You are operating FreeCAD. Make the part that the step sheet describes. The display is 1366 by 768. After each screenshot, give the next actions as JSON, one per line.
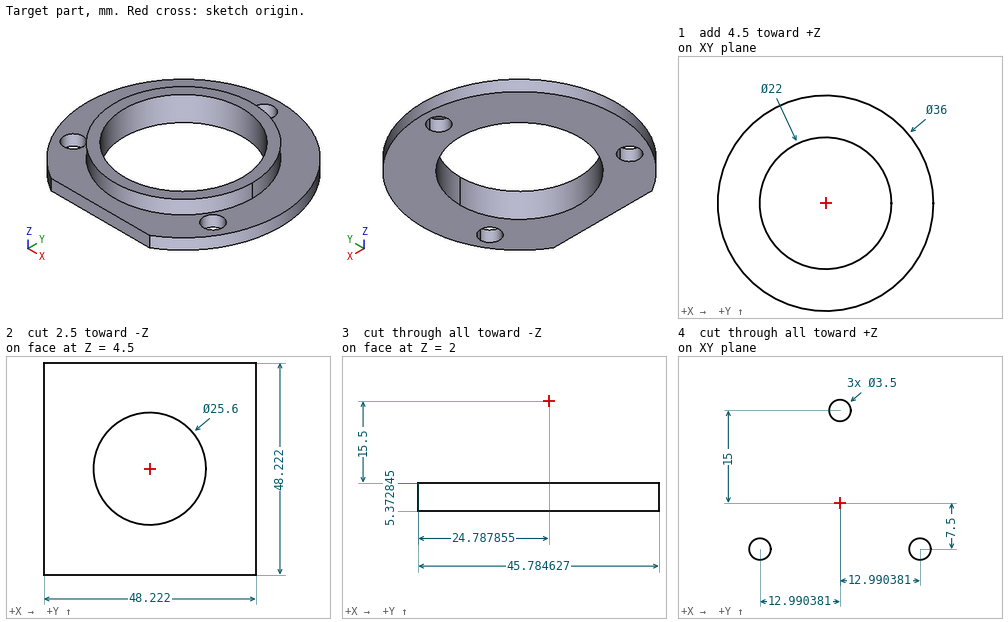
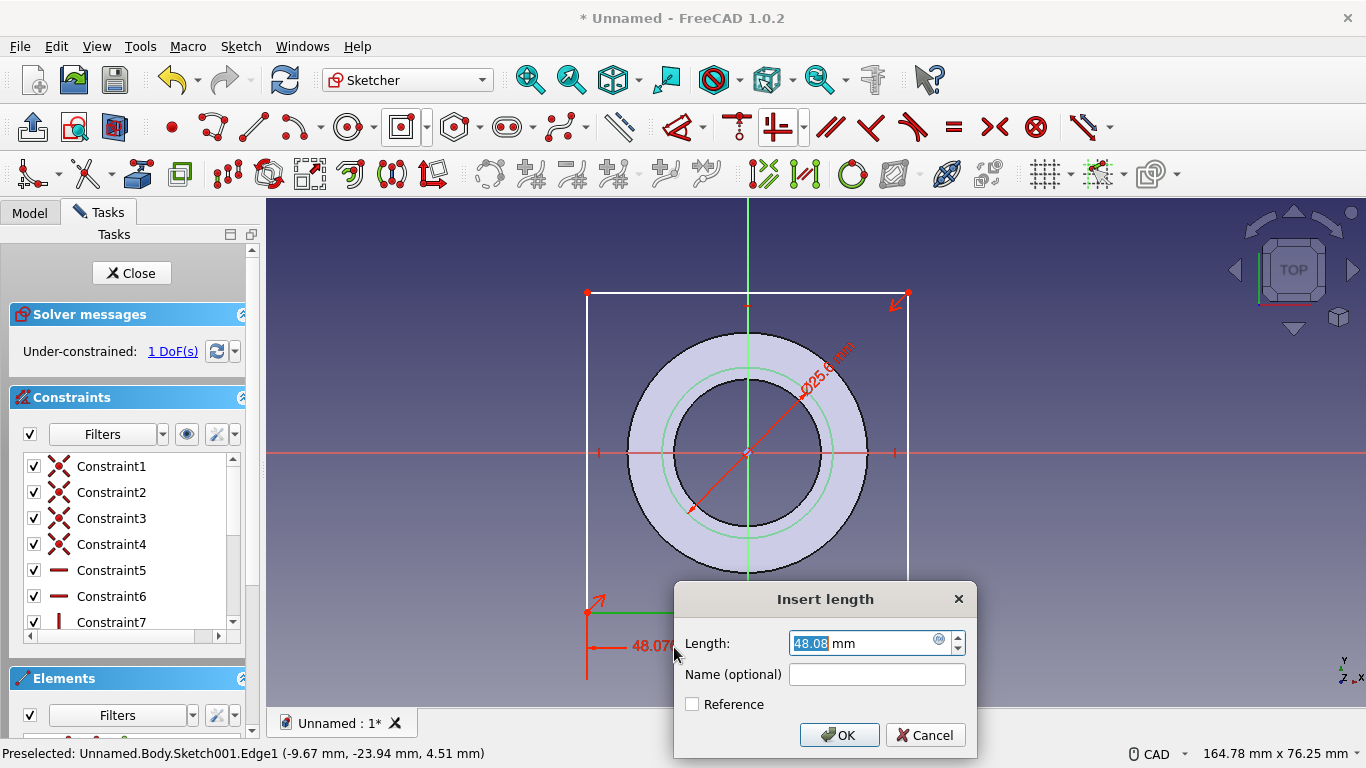
{"action": "type", "text": "48.222"}
{"action": "key", "text": "Return"}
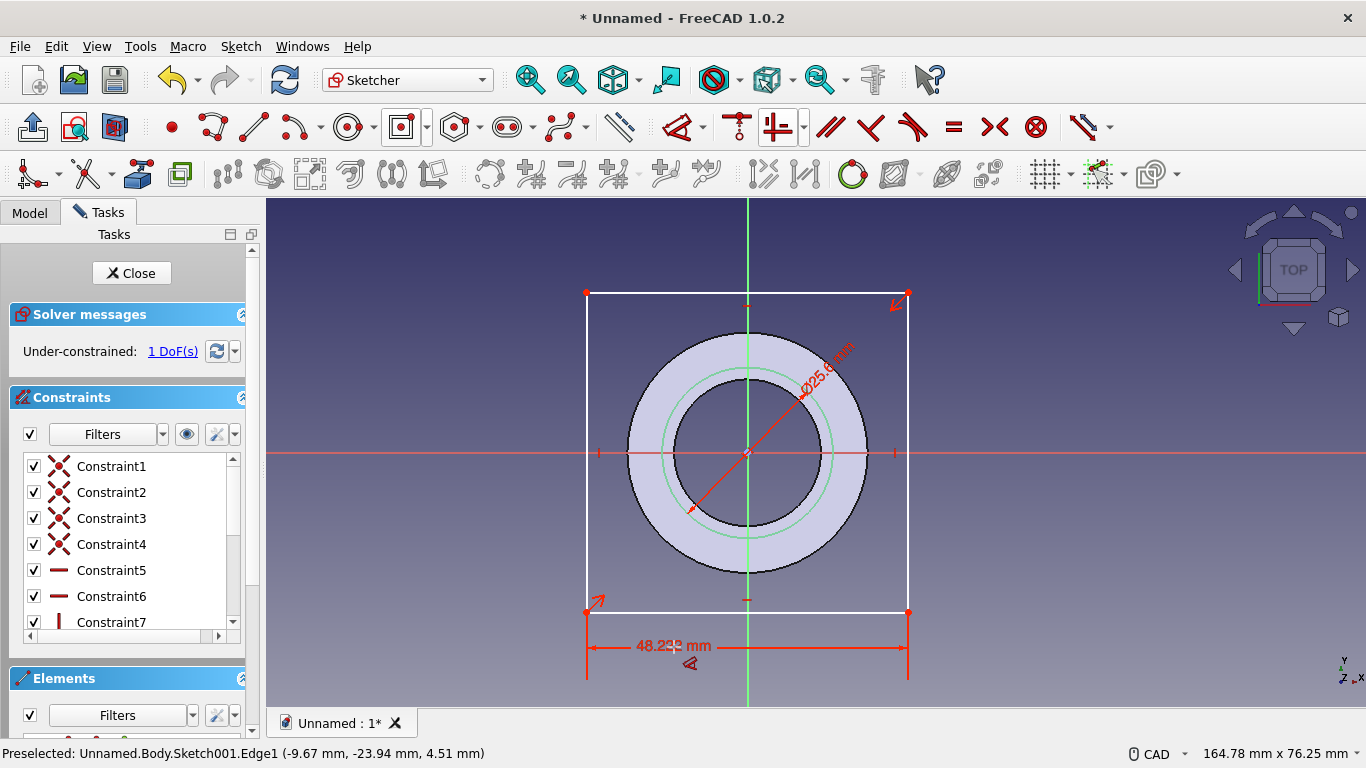
{"action": "left_click", "coordinate": [908, 517]}
{"action": "left_click", "coordinate": [942, 379]}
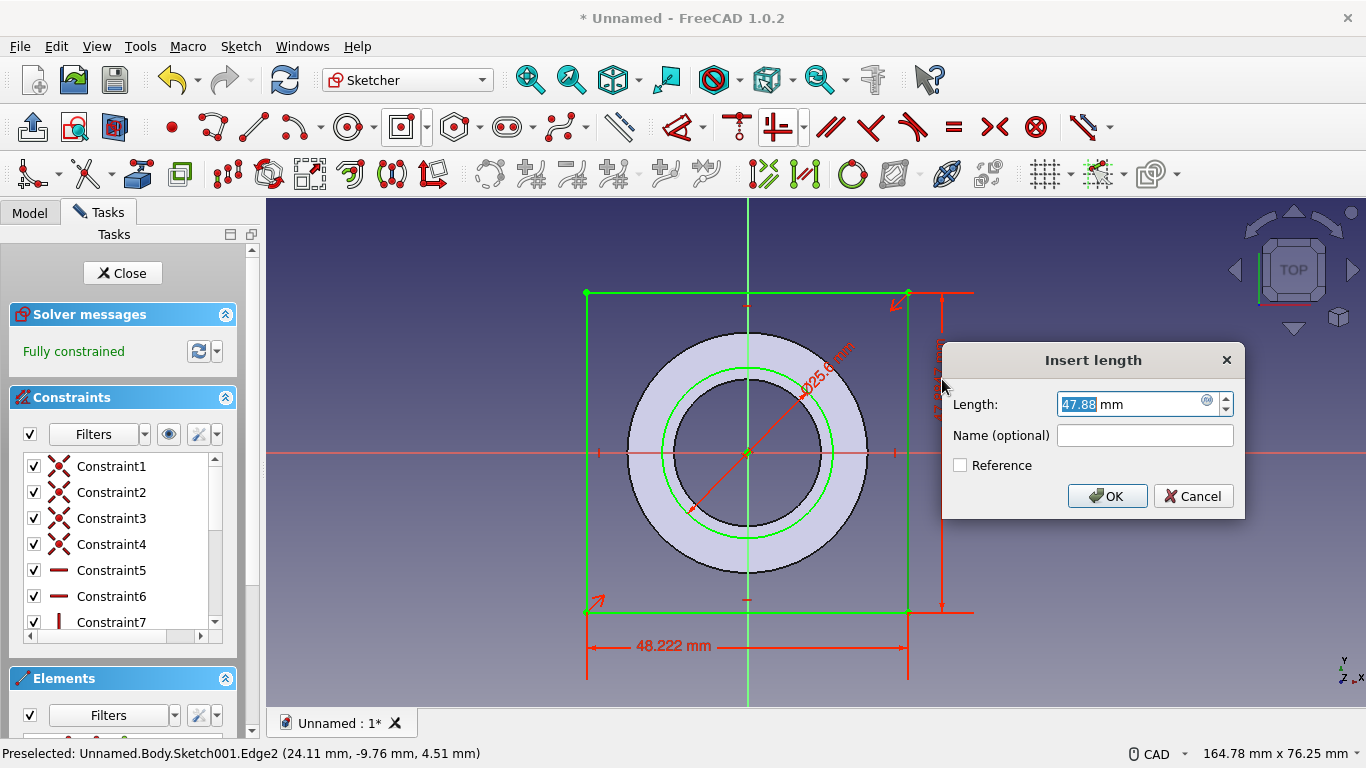
{"action": "type", "text": "48.222"}
{"action": "key", "text": "Return"}
{"action": "key", "text": "Escape"}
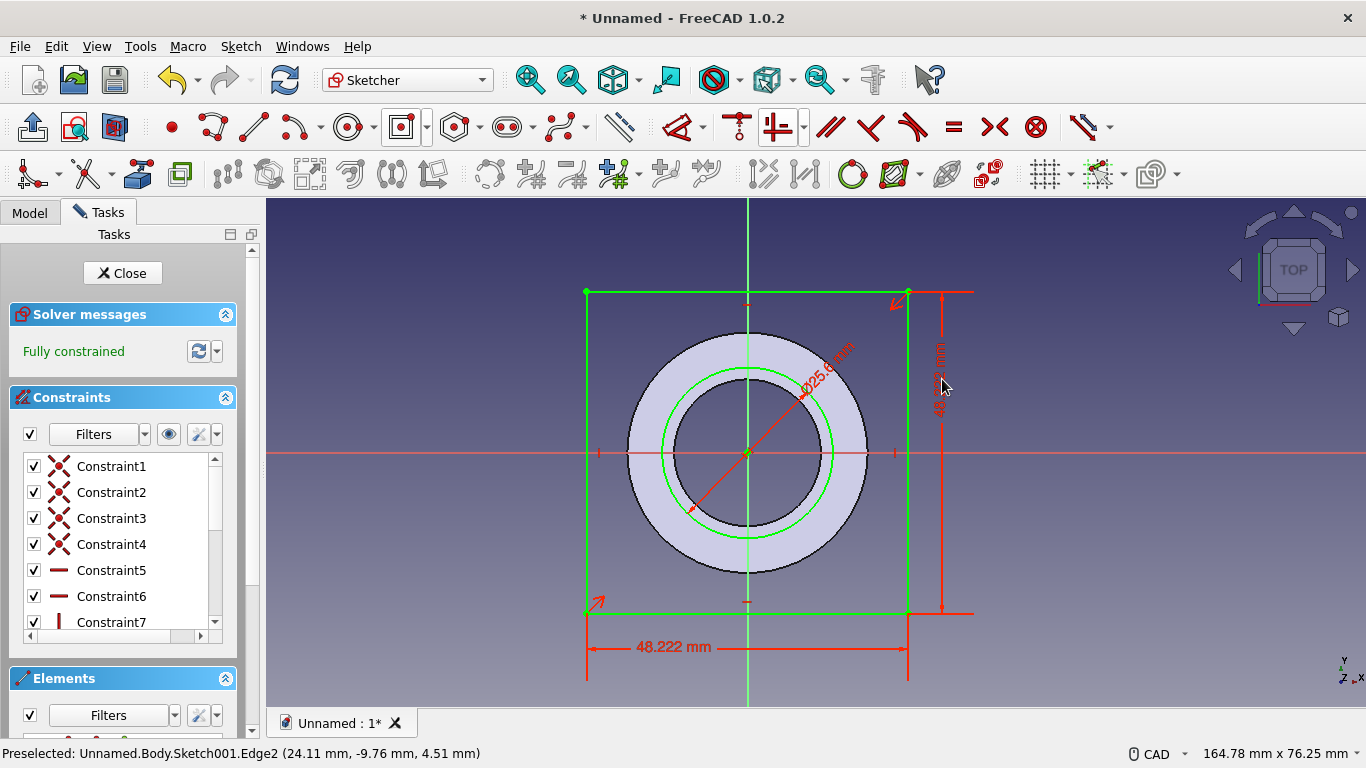
{"action": "left_click", "coordinate": [123, 273]}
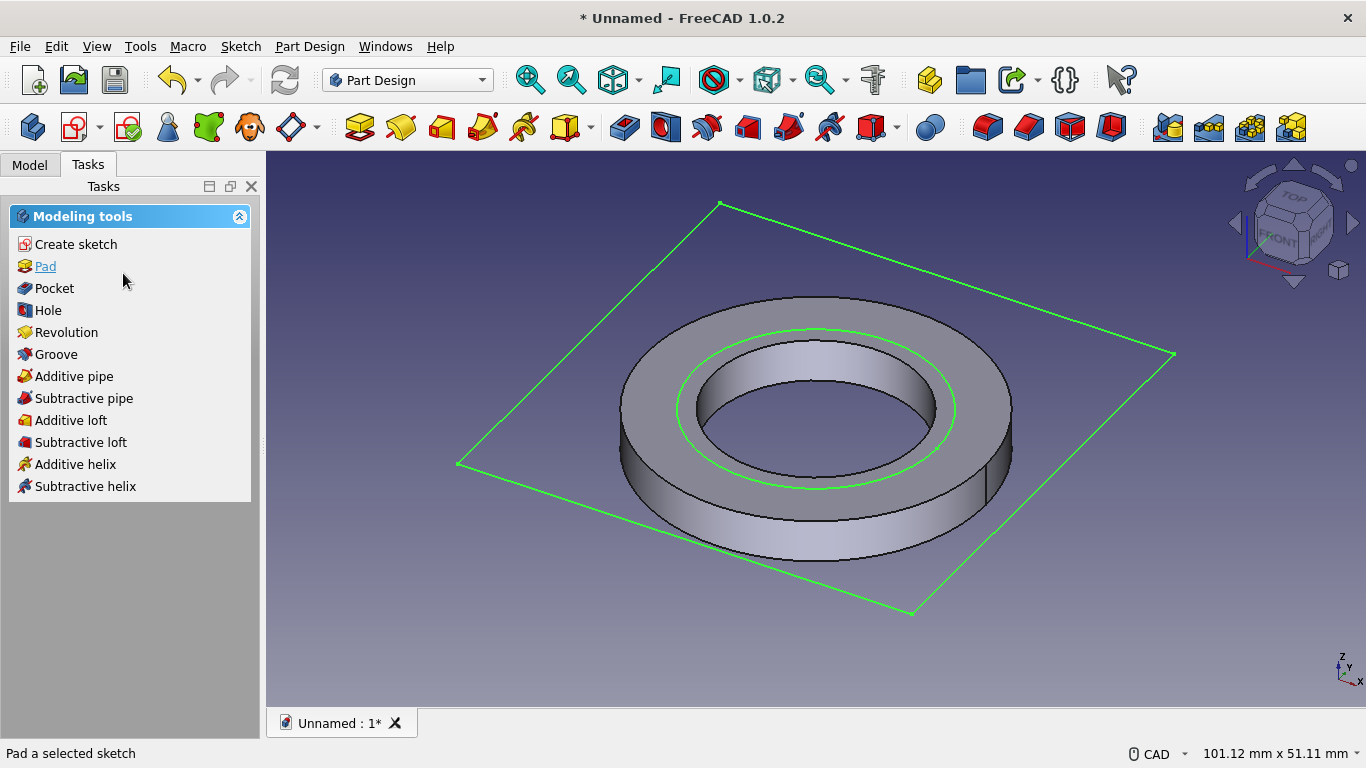
{"action": "left_click", "coordinate": [625, 128]}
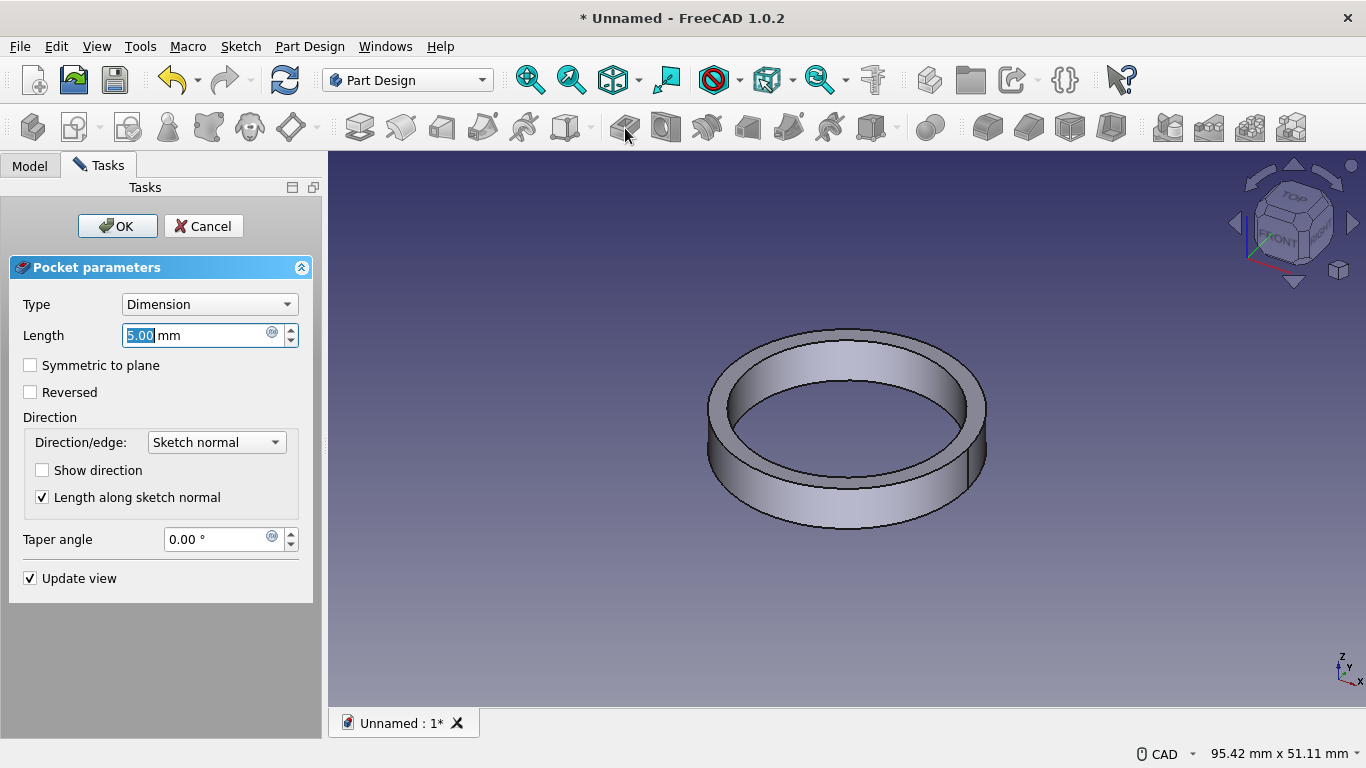
{"action": "type", "text": "2.5"}
{"action": "key", "text": "Tab"}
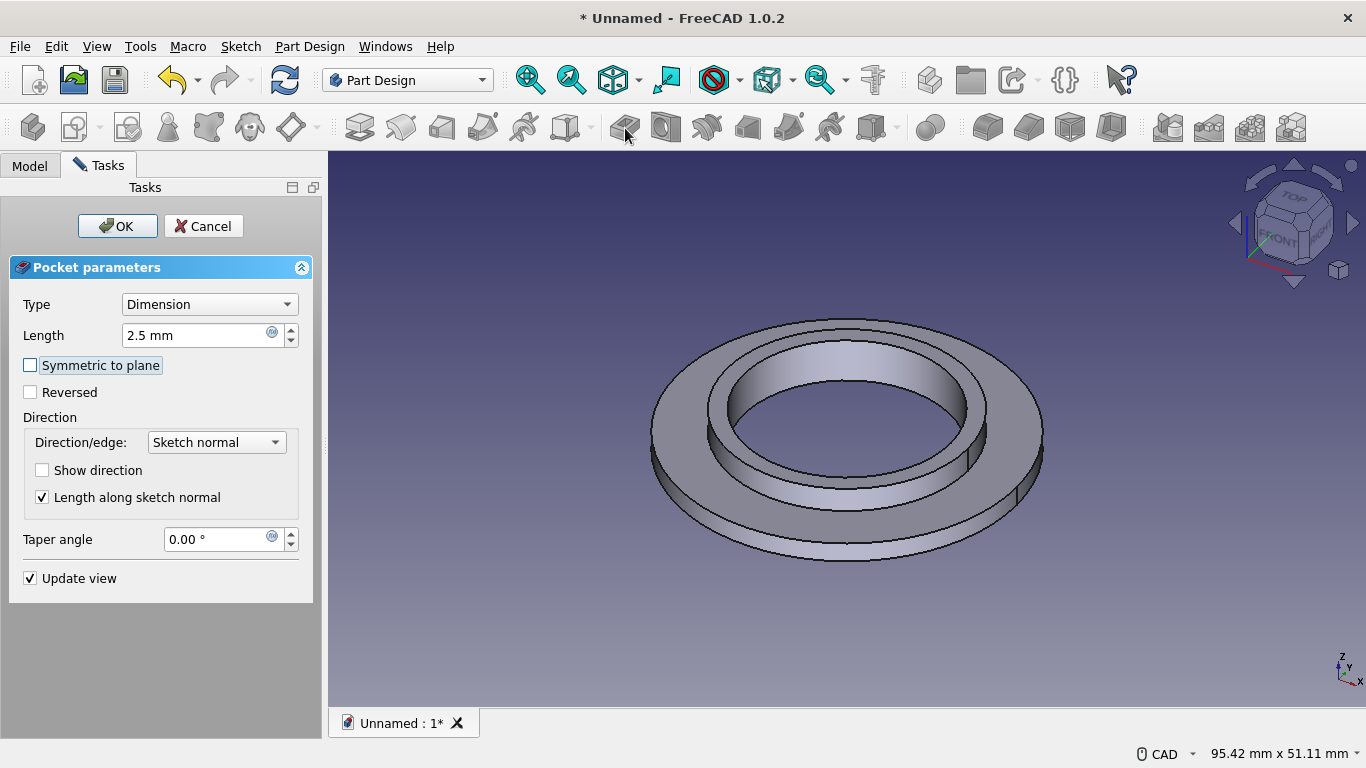
{"action": "left_click", "coordinate": [118, 226]}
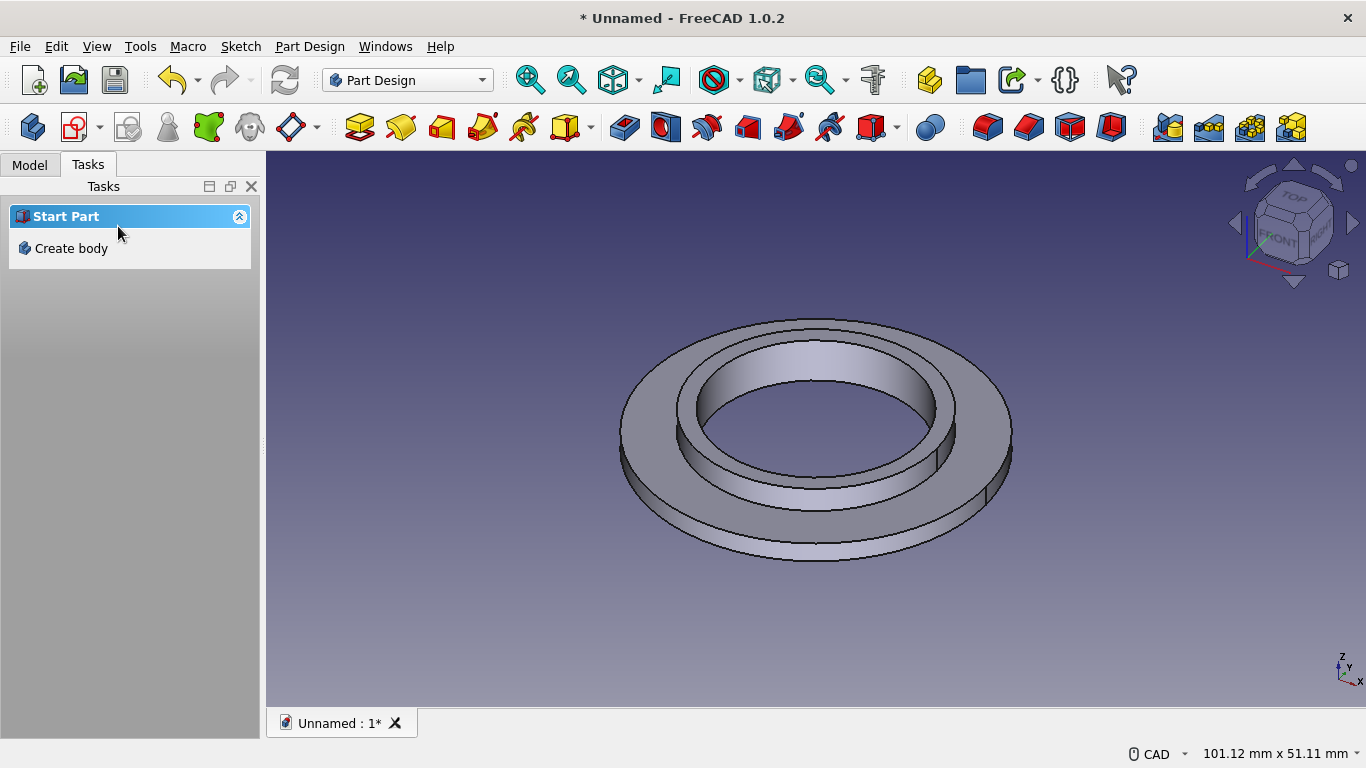
{"action": "left_click", "coordinate": [732, 514]}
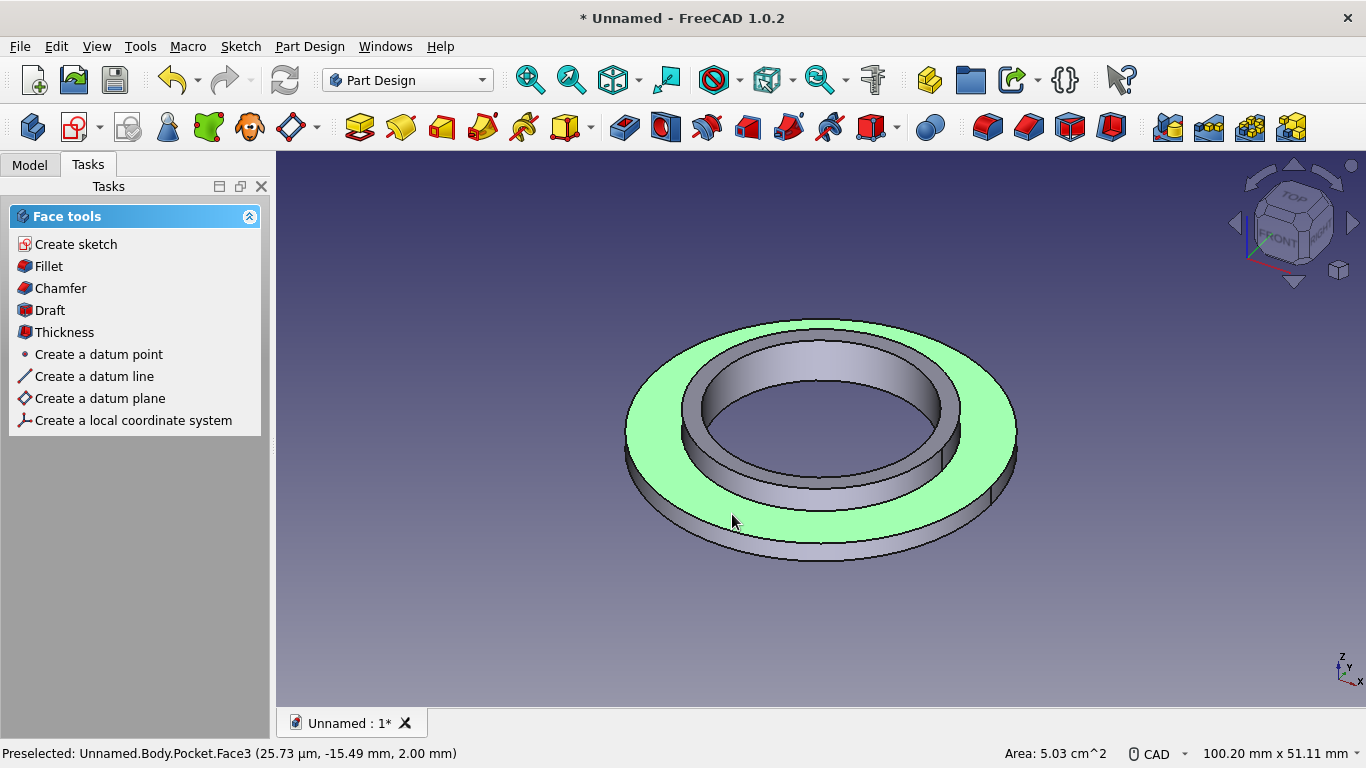
{"action": "left_click", "coordinate": [74, 128]}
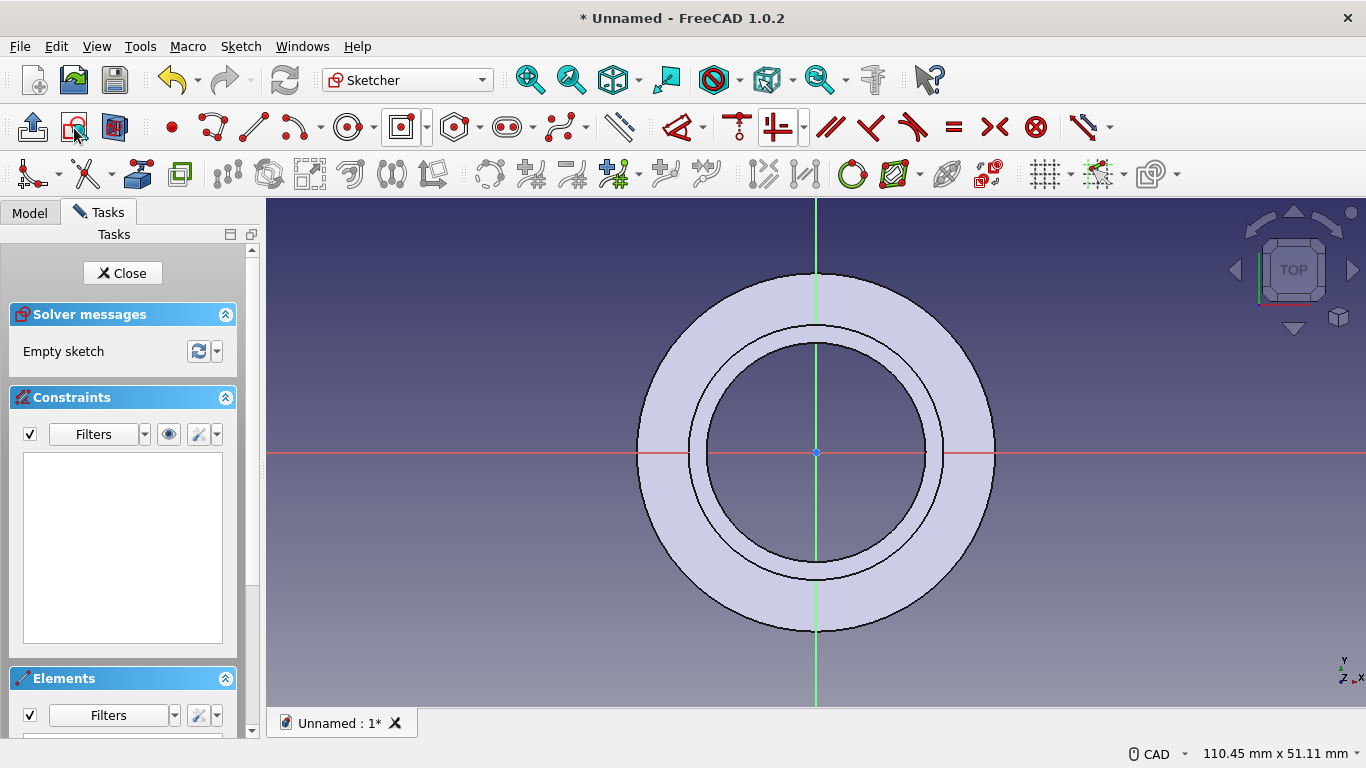
{"action": "scroll", "coordinate": [898, 679], "scroll_direction": "up", "scroll_amount": 2}